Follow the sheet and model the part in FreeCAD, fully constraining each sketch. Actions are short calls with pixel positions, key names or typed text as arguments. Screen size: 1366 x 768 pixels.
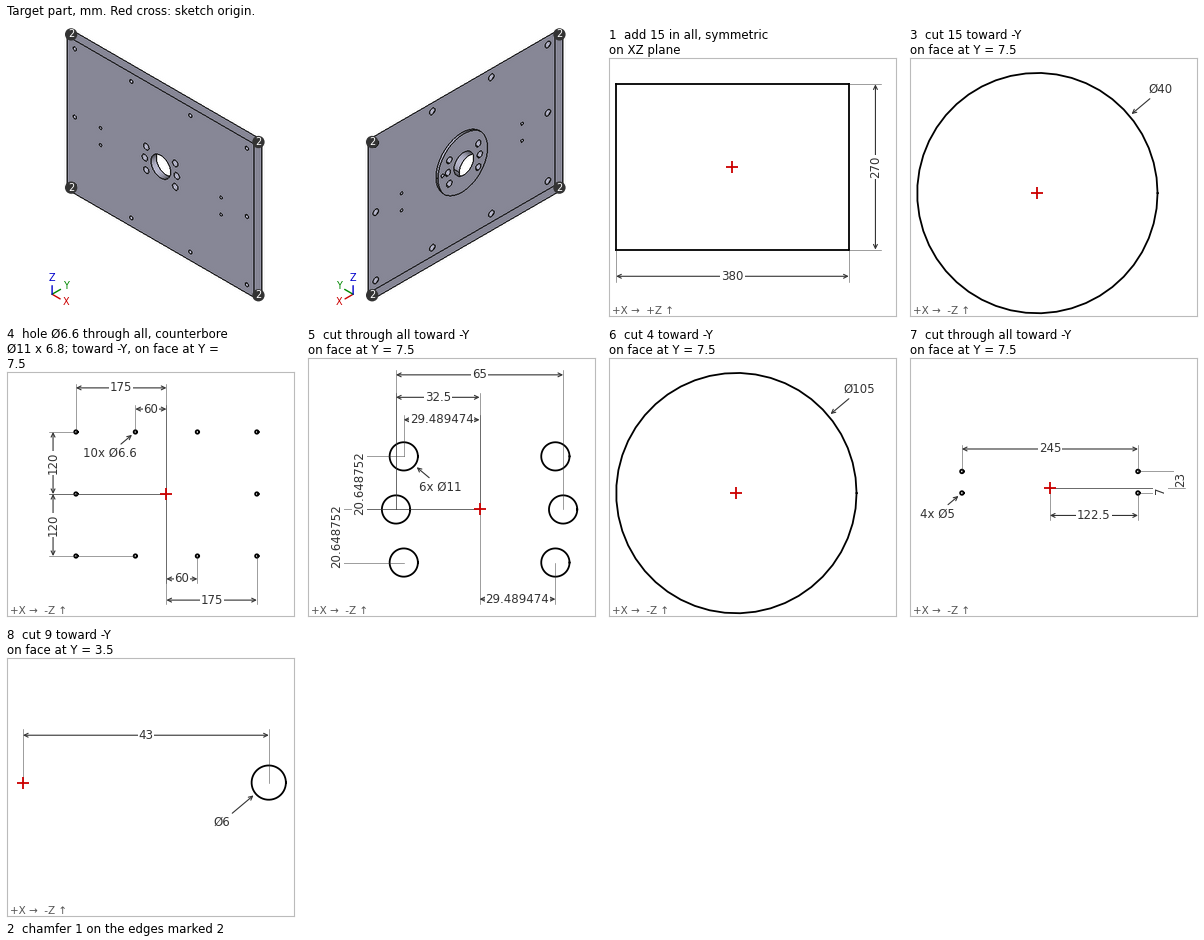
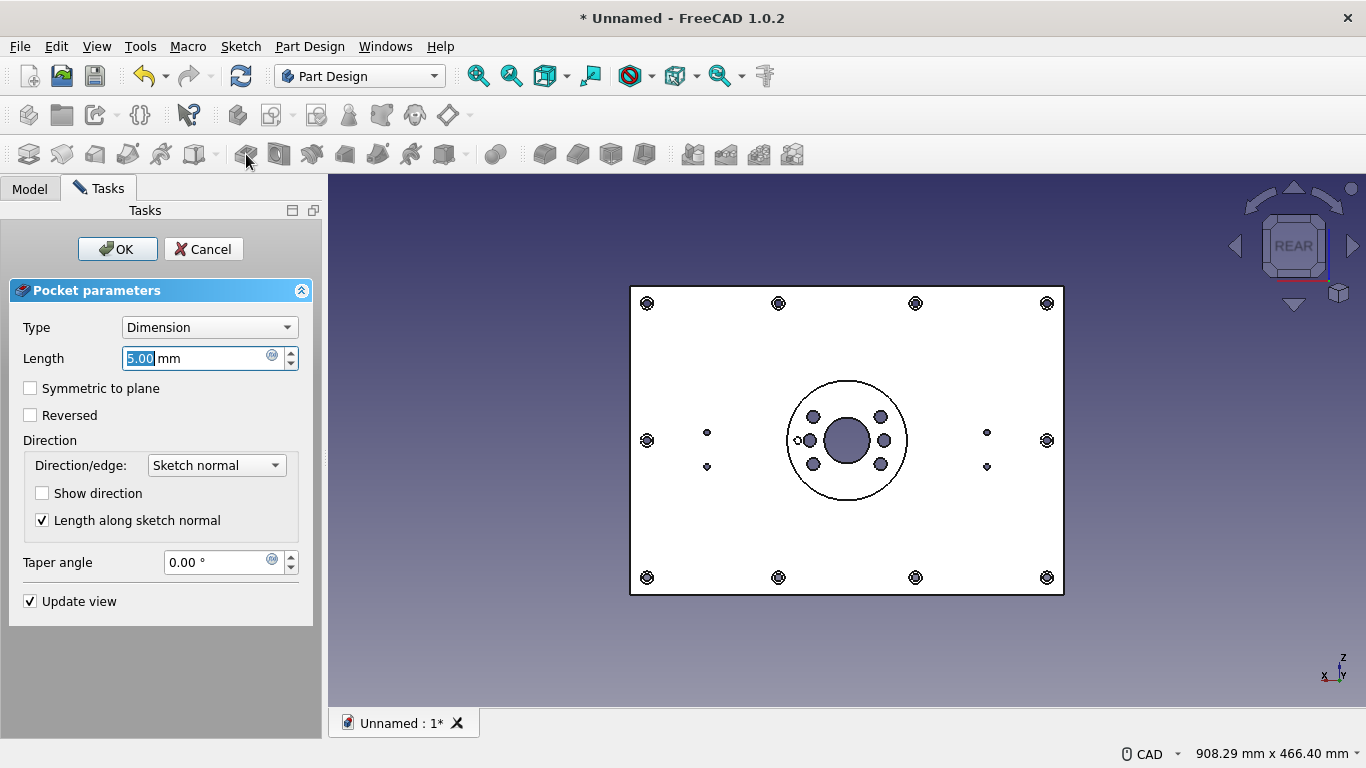
text(9)
key(Tab)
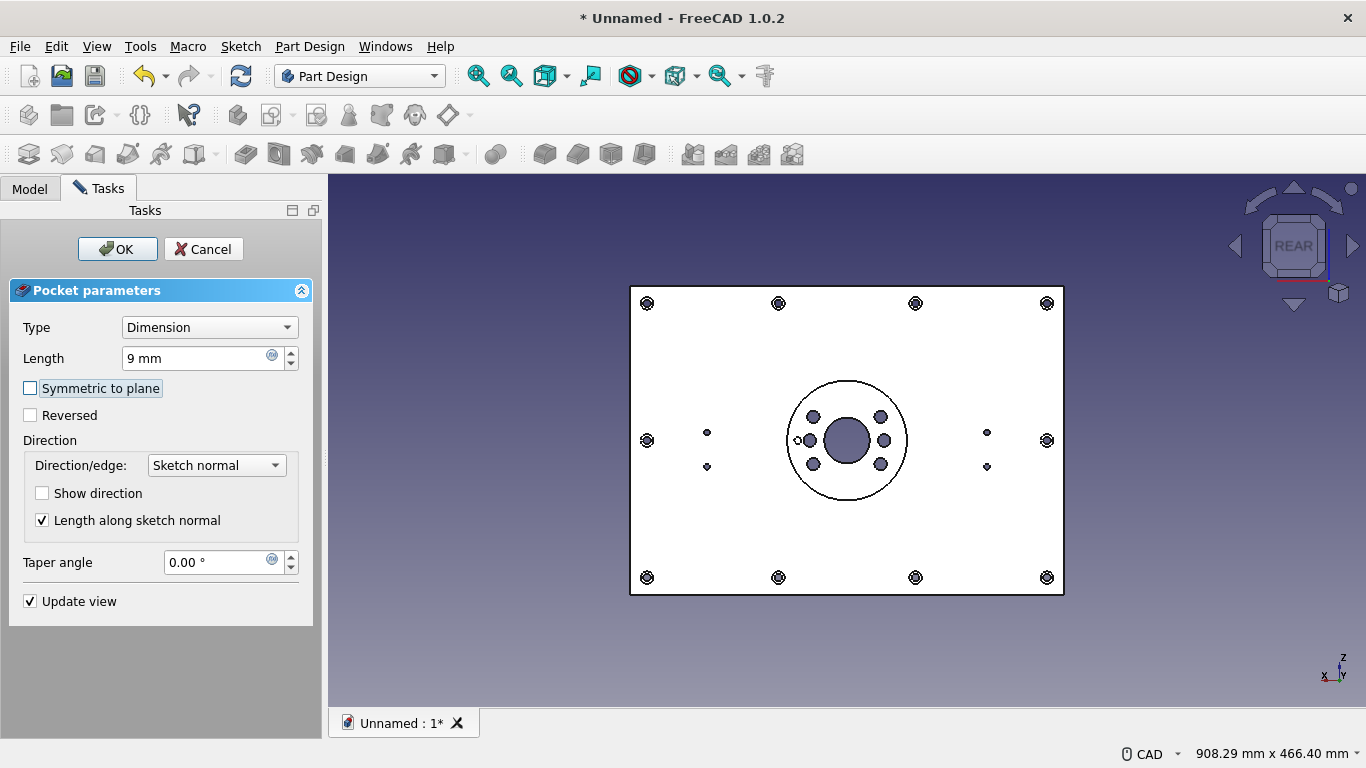
click(118, 249)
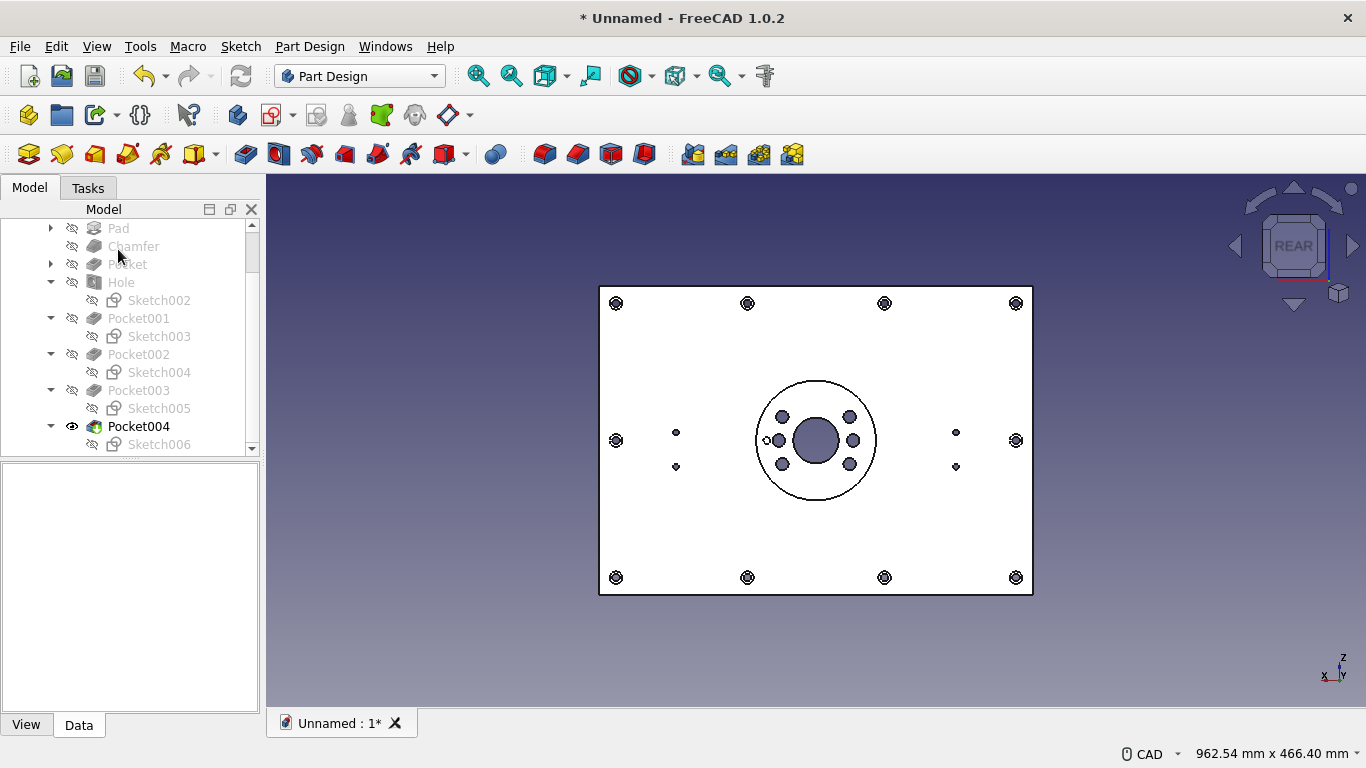
key(0)